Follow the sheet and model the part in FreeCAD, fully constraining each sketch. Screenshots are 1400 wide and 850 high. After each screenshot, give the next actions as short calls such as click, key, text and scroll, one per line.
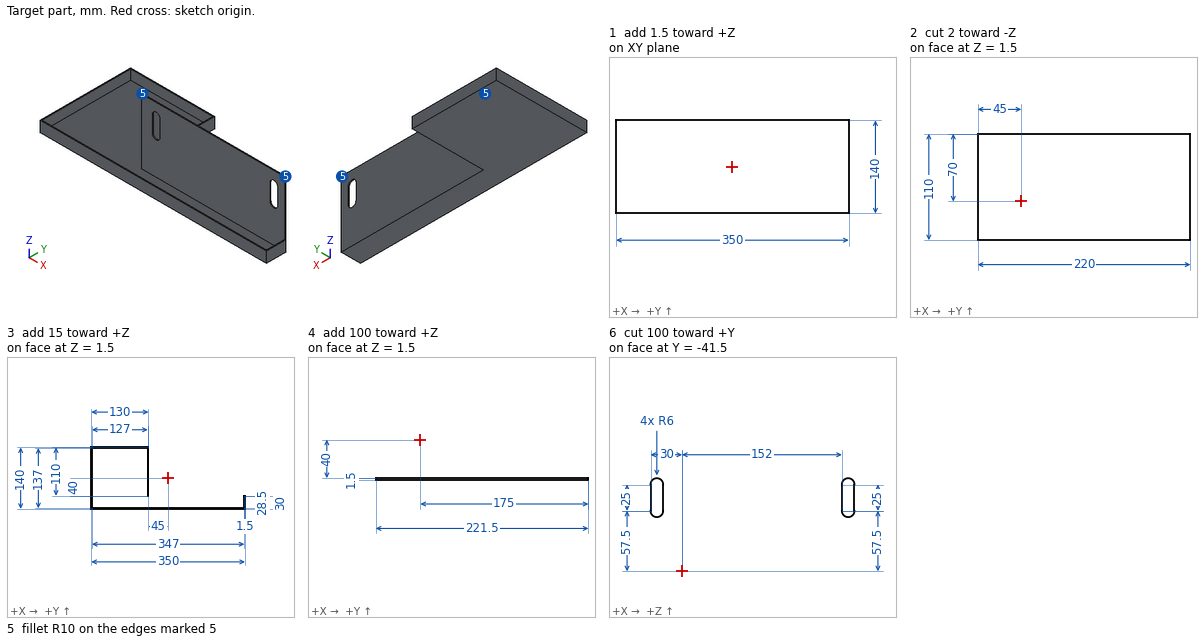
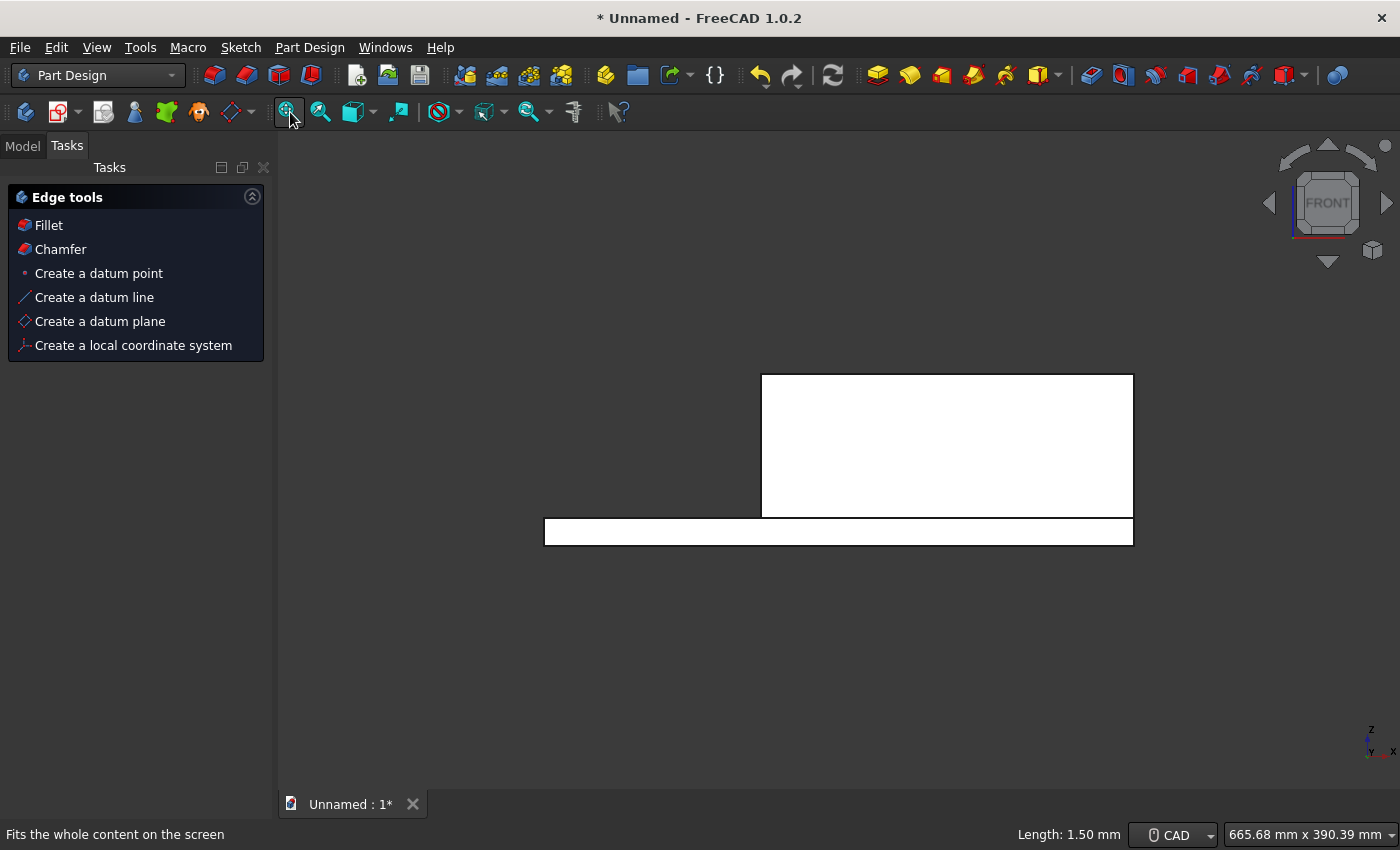
key(3)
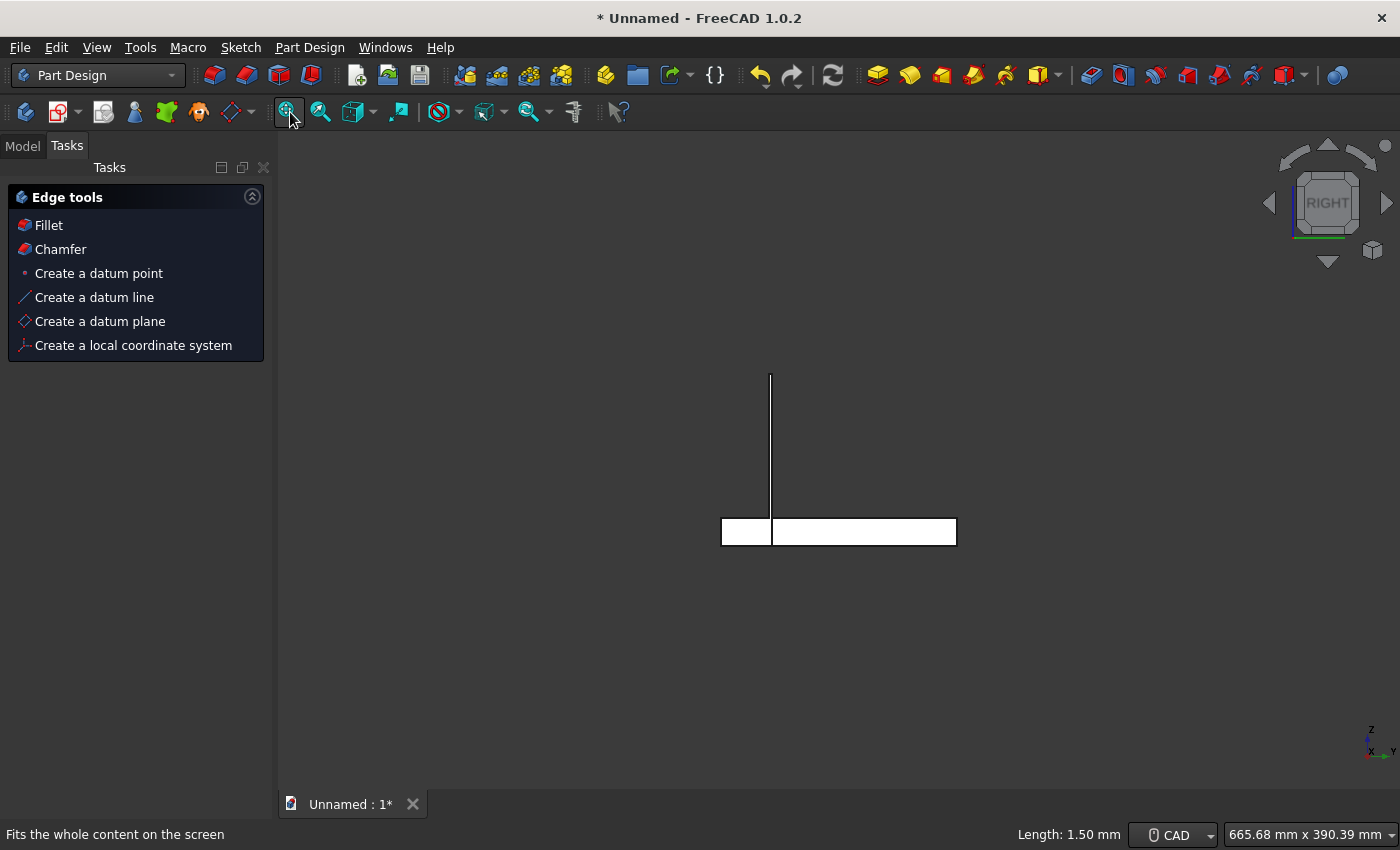
click(290, 112)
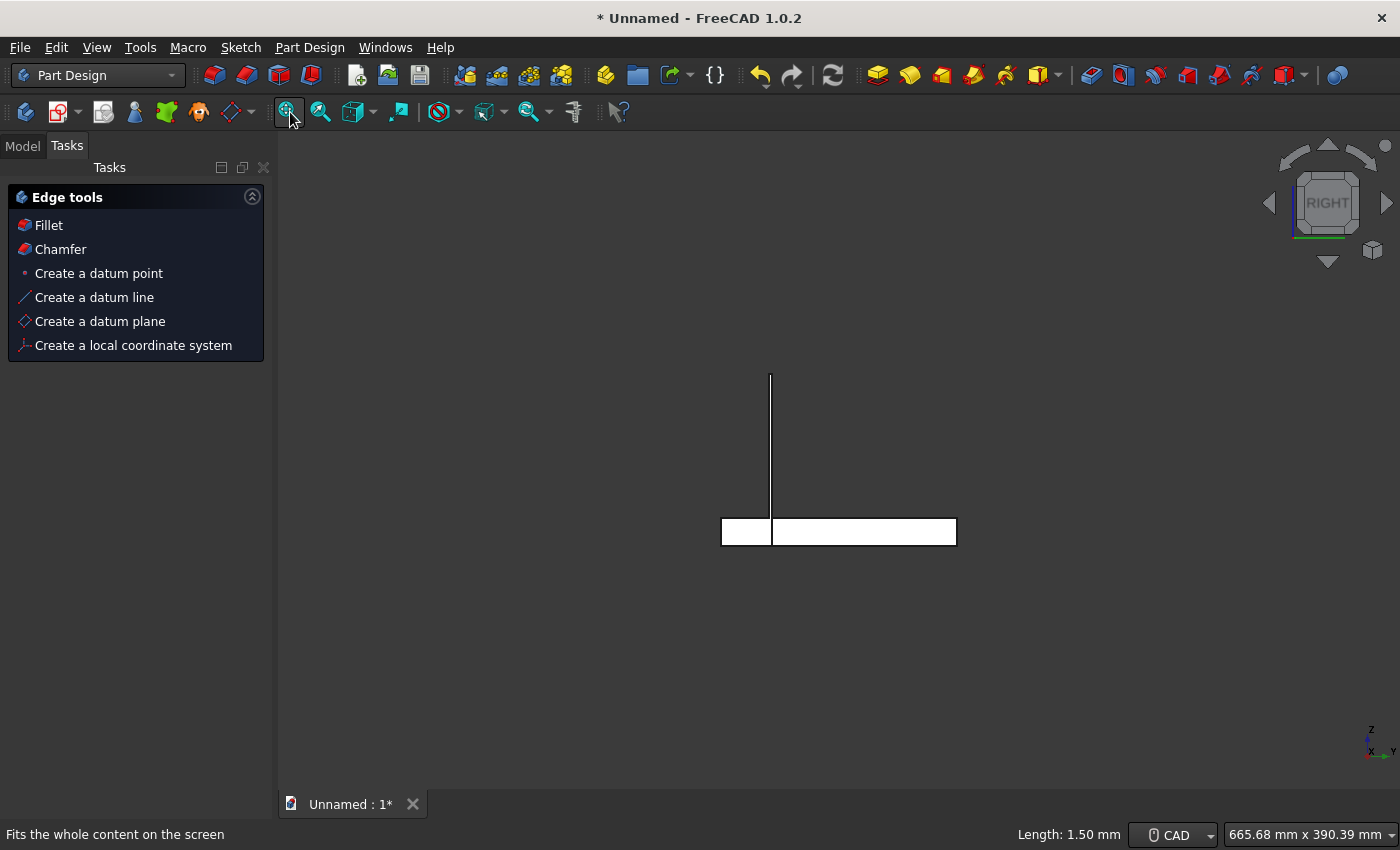
scroll(770, 373, up, 14)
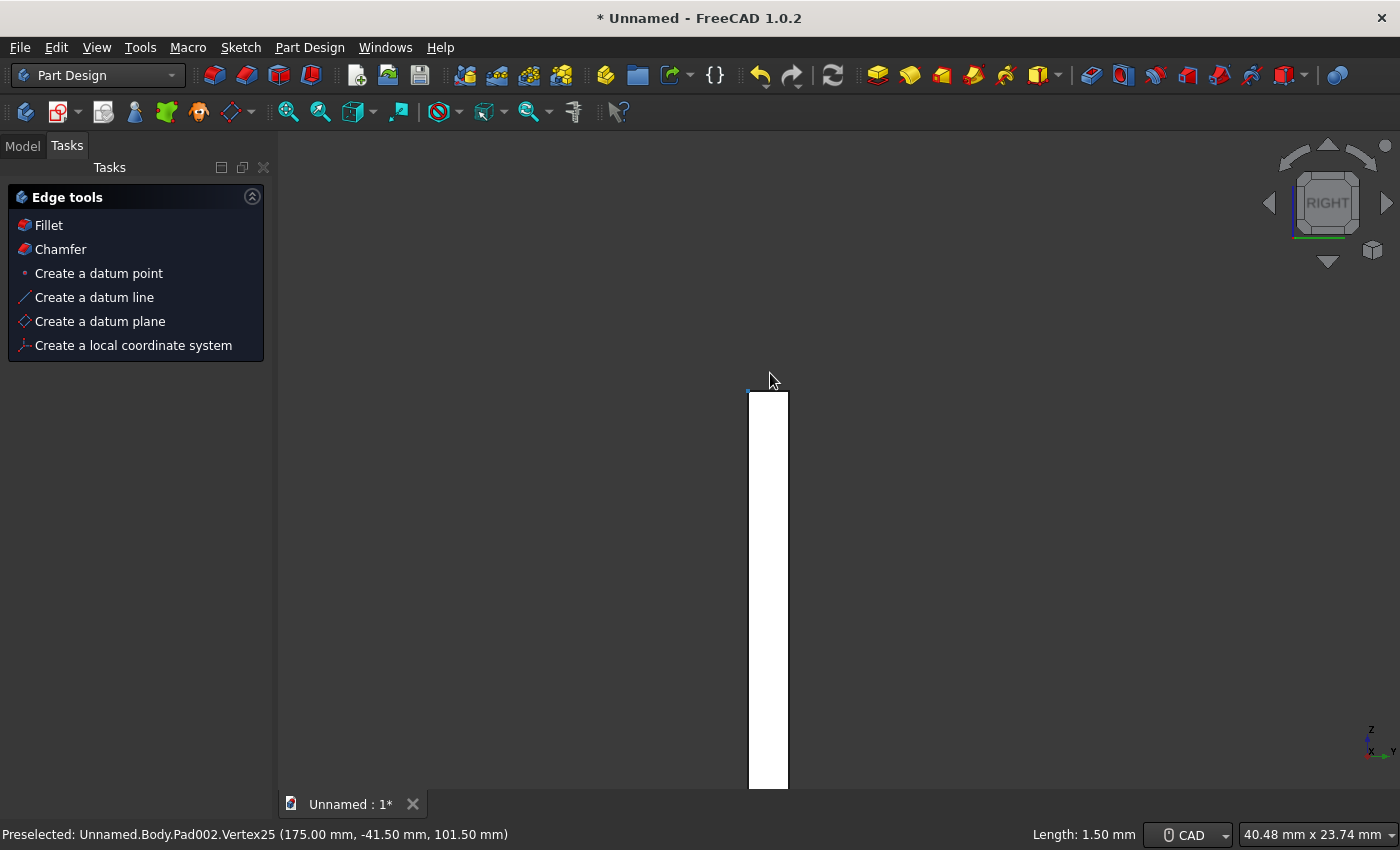
click(768, 390, ctrl)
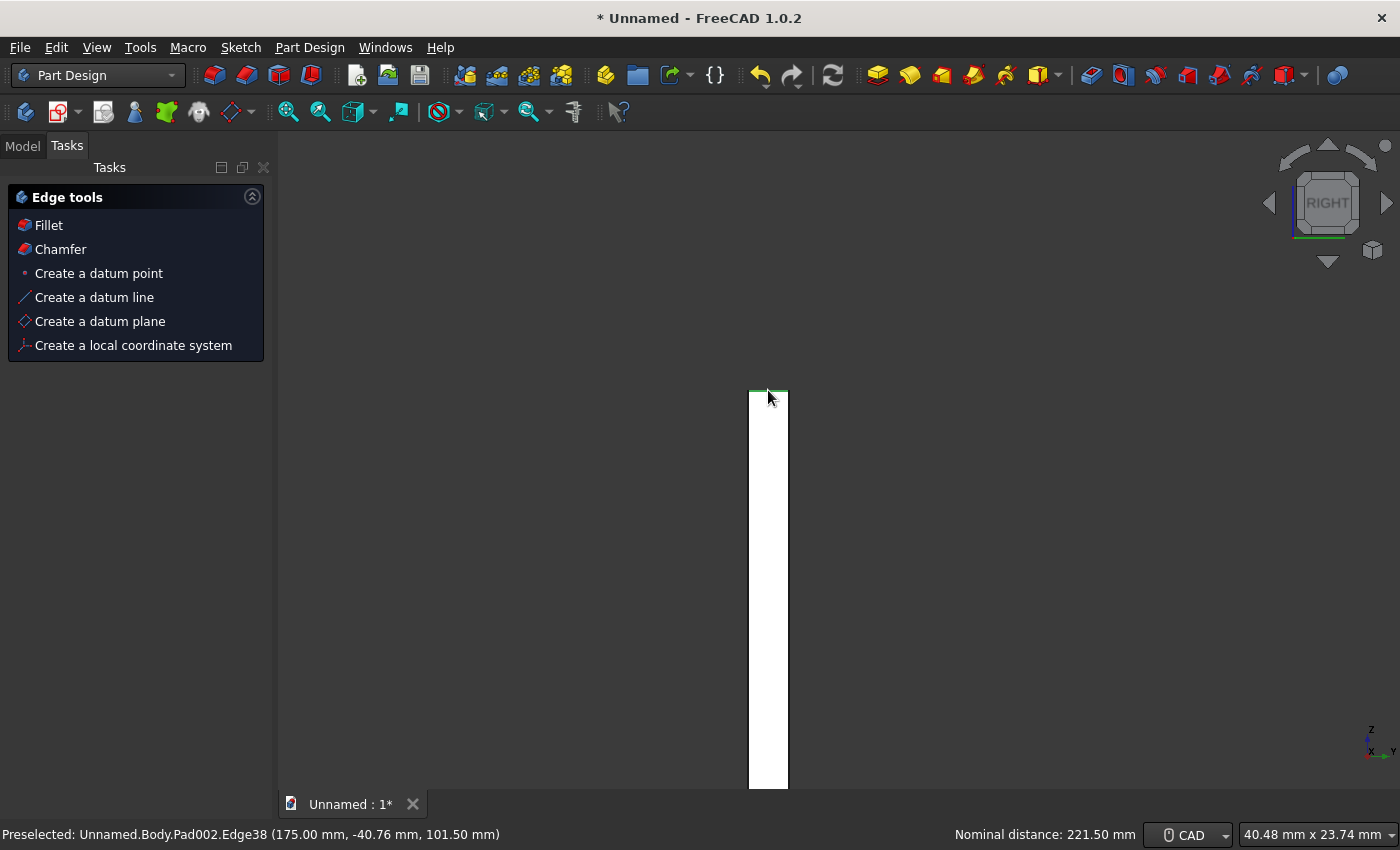
click(216, 76)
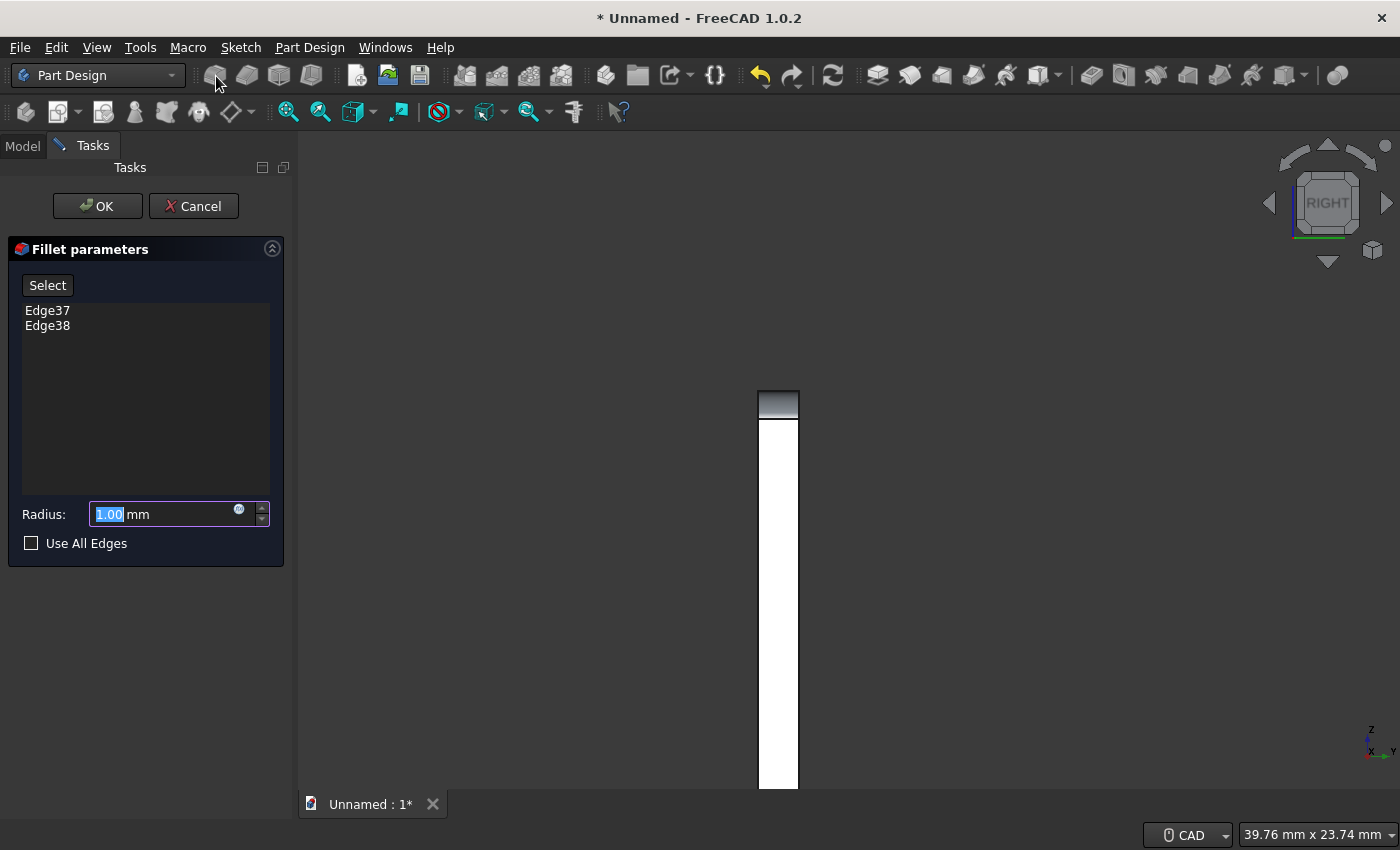
text(10)
key(Tab)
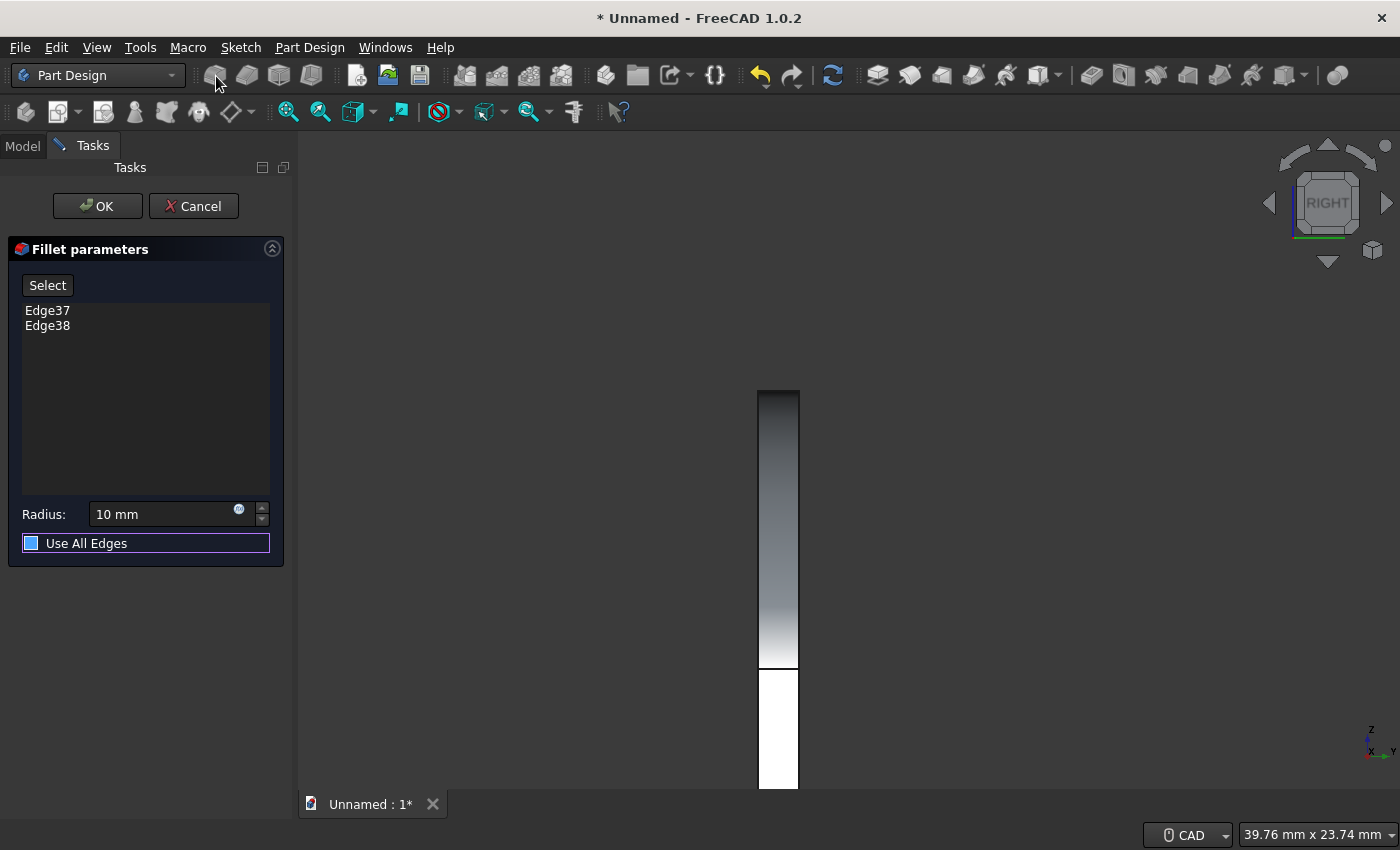
click(98, 206)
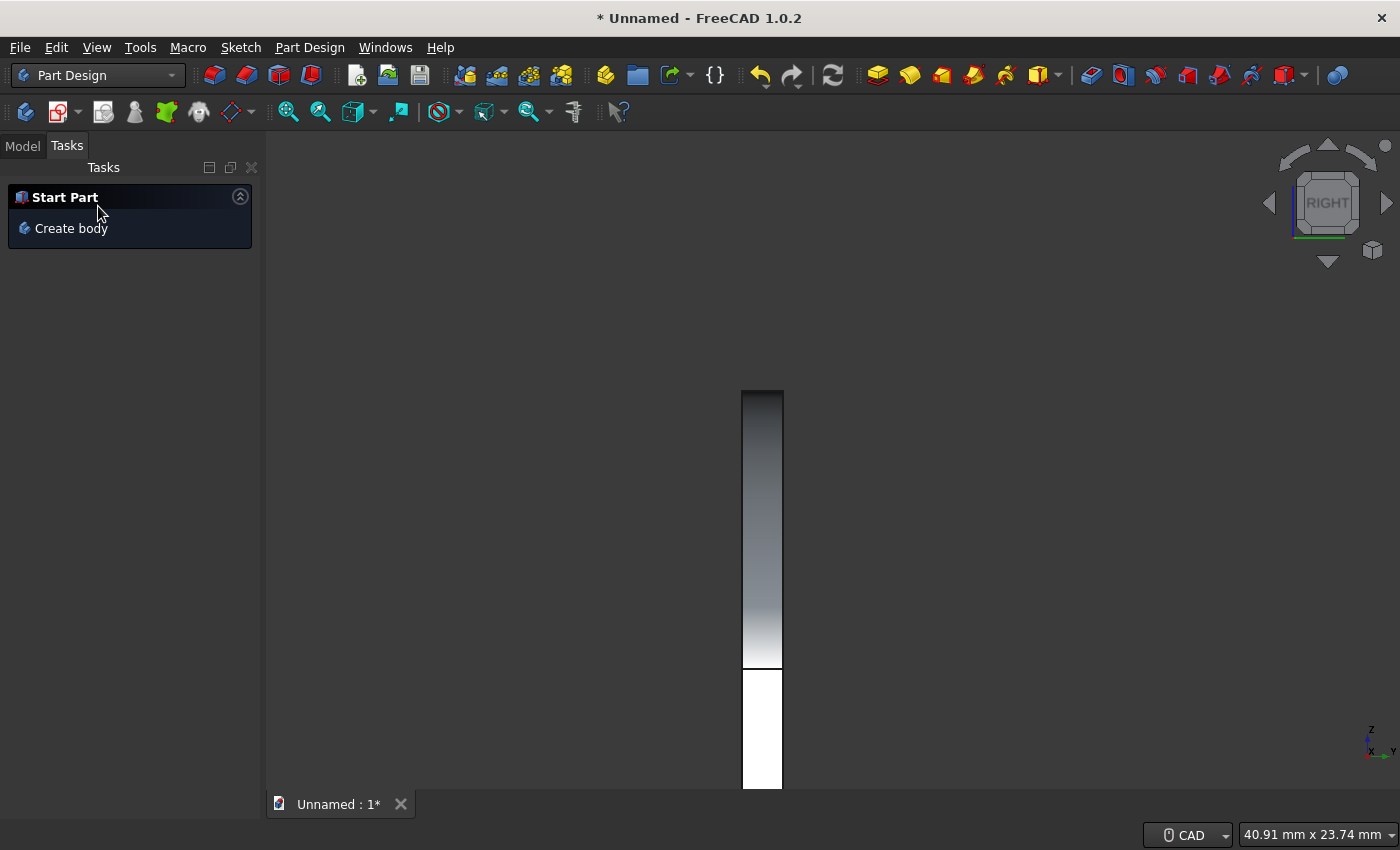
click(290, 112)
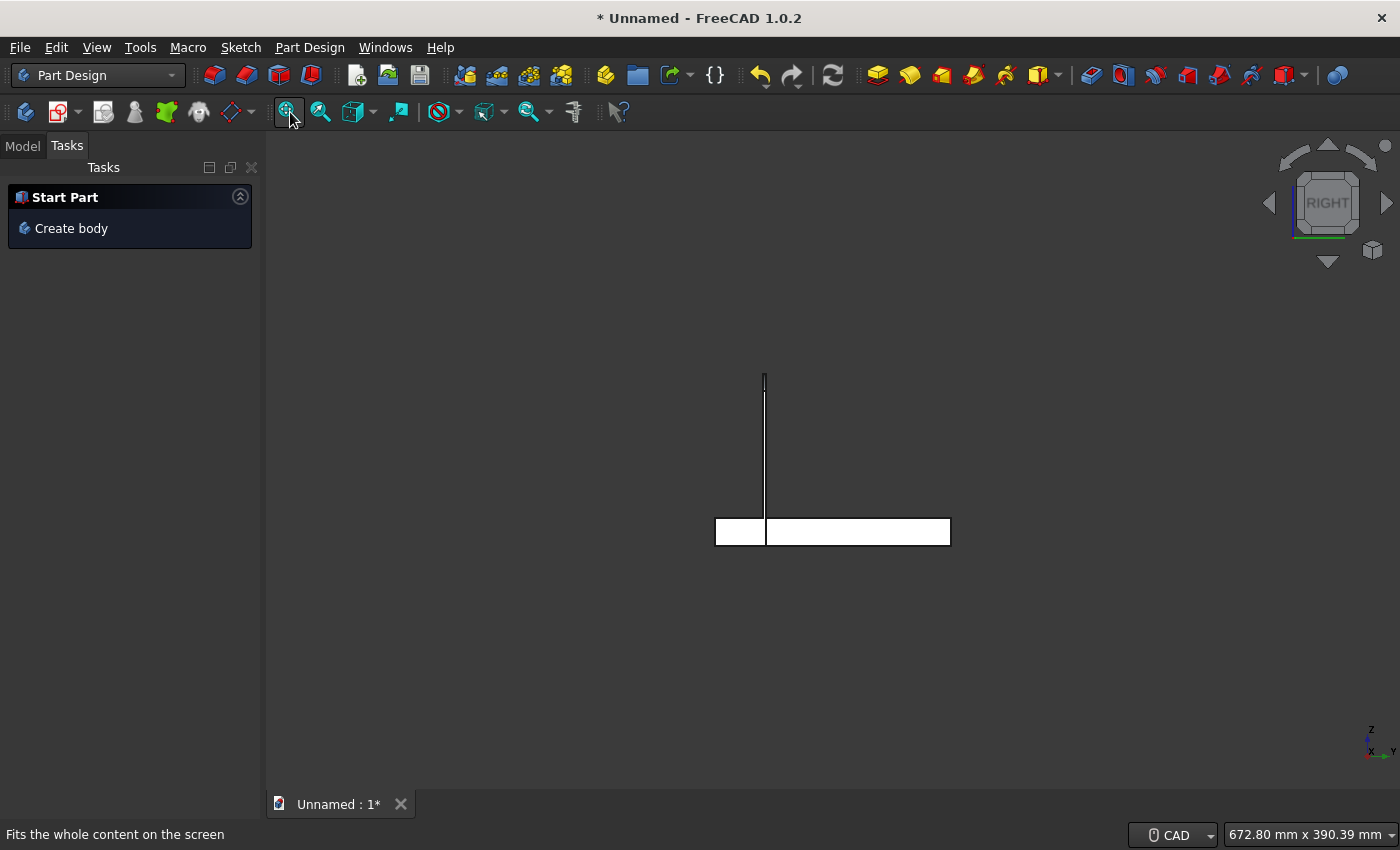
key(0)